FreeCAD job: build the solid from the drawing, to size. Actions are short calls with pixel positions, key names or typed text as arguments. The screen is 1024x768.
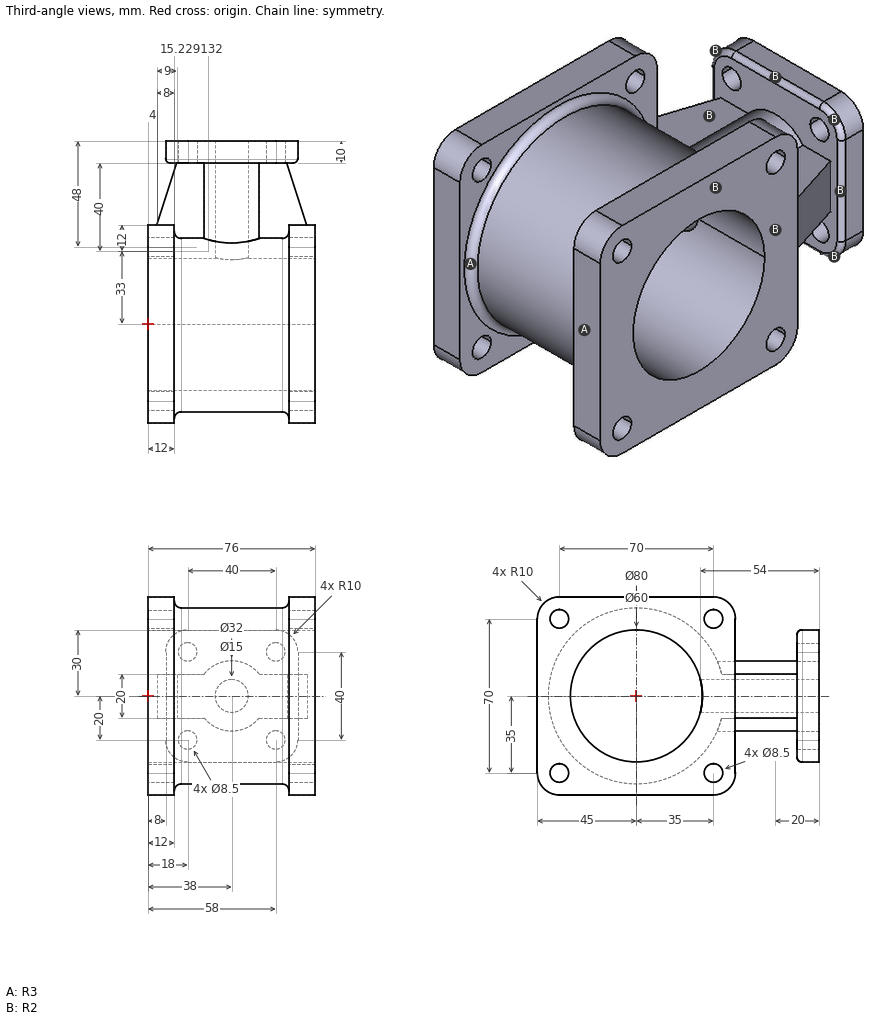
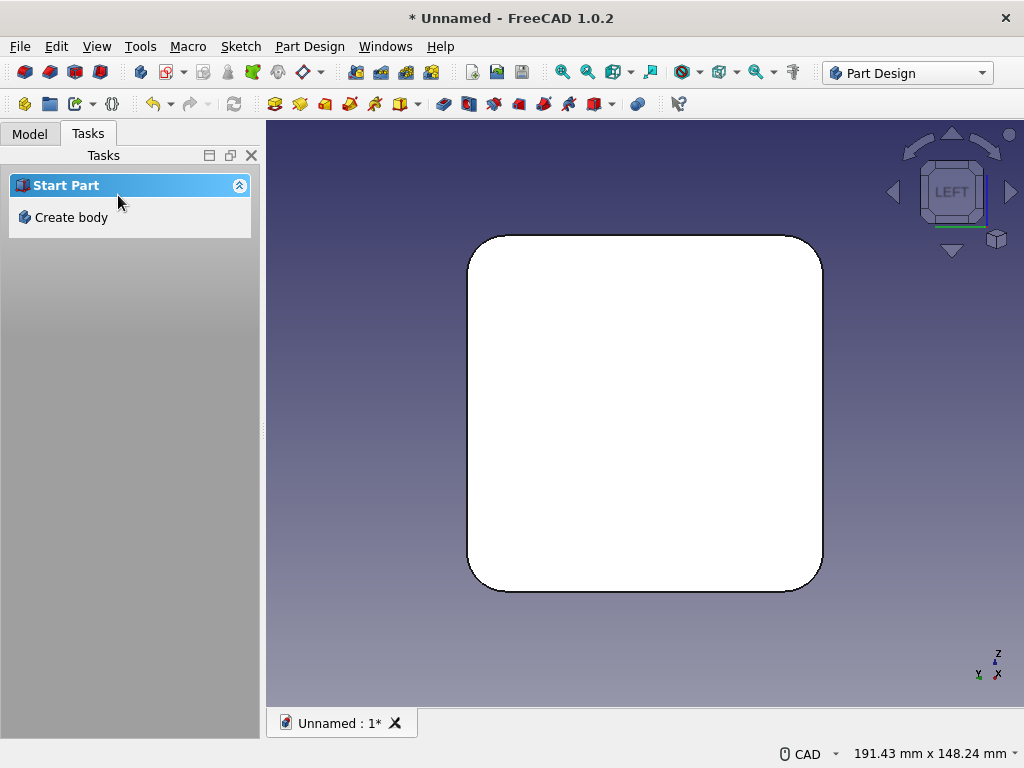
click(645, 412)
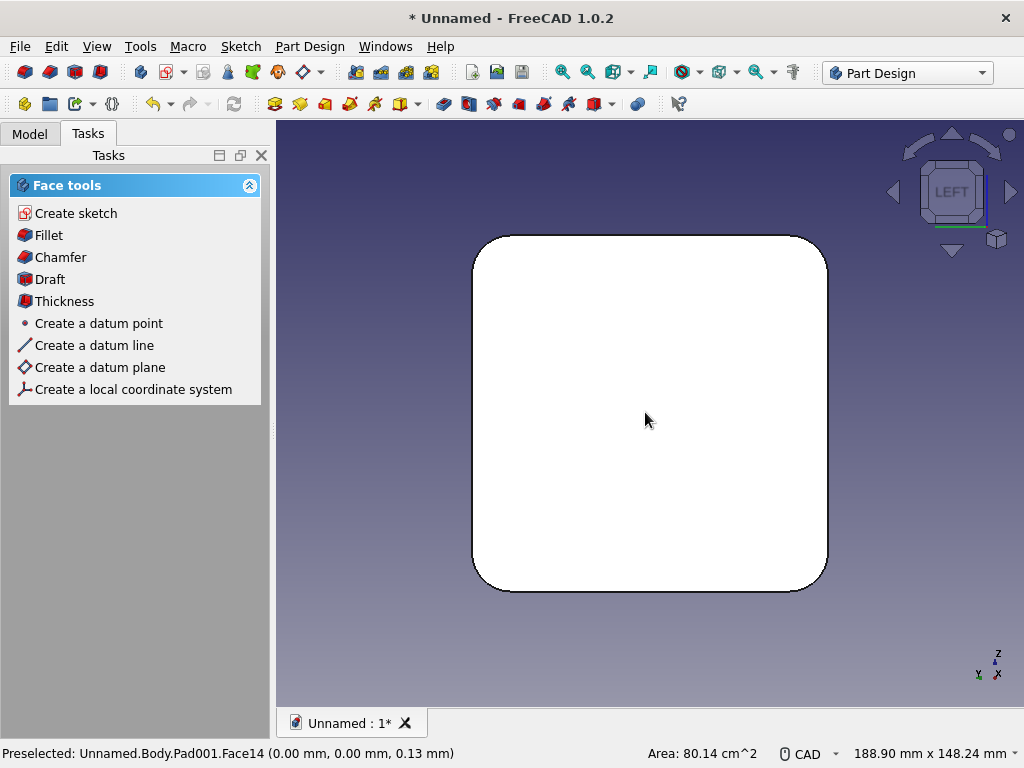
click(166, 72)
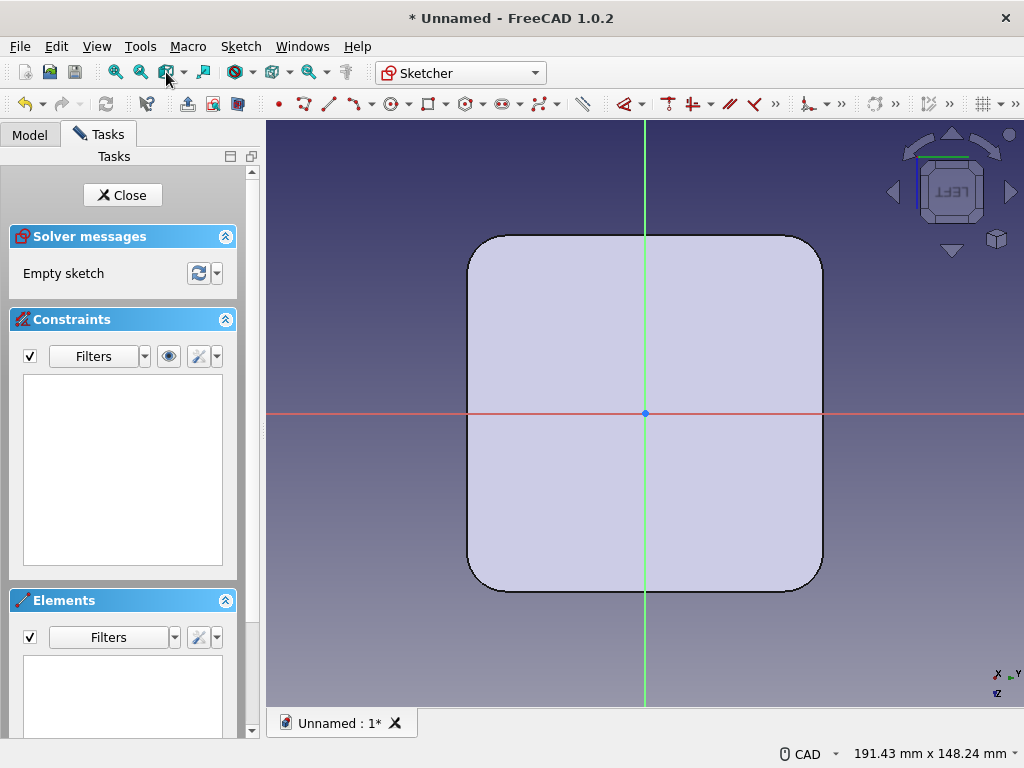
scroll(784, 413, up, 2)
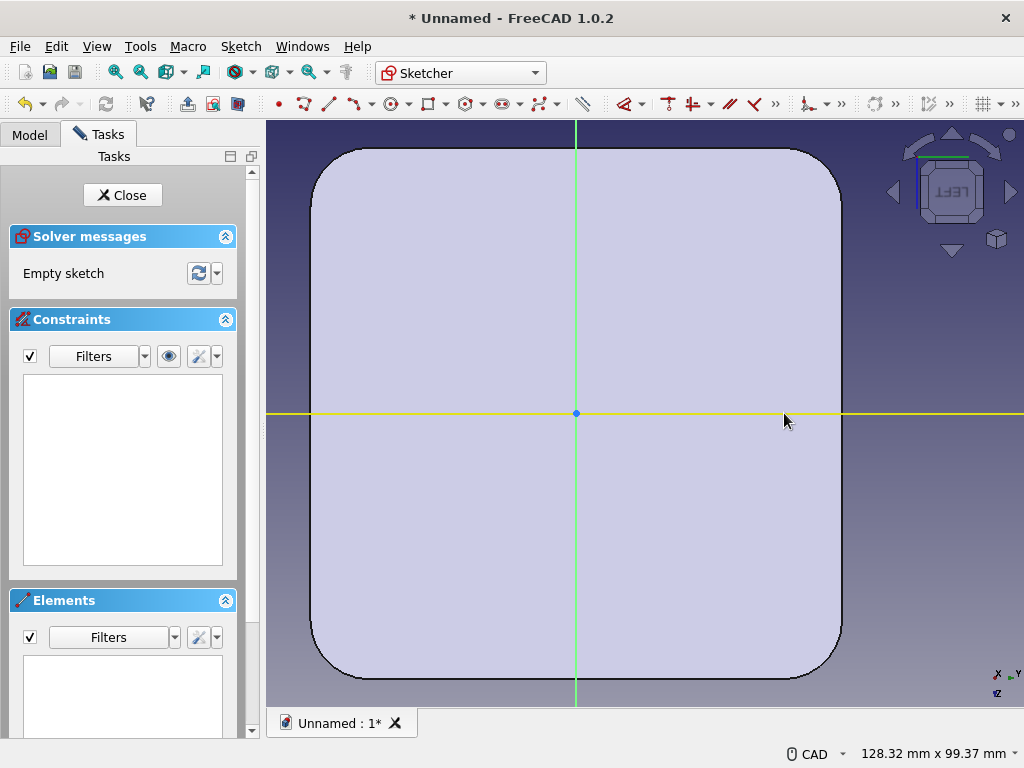
click(390, 104)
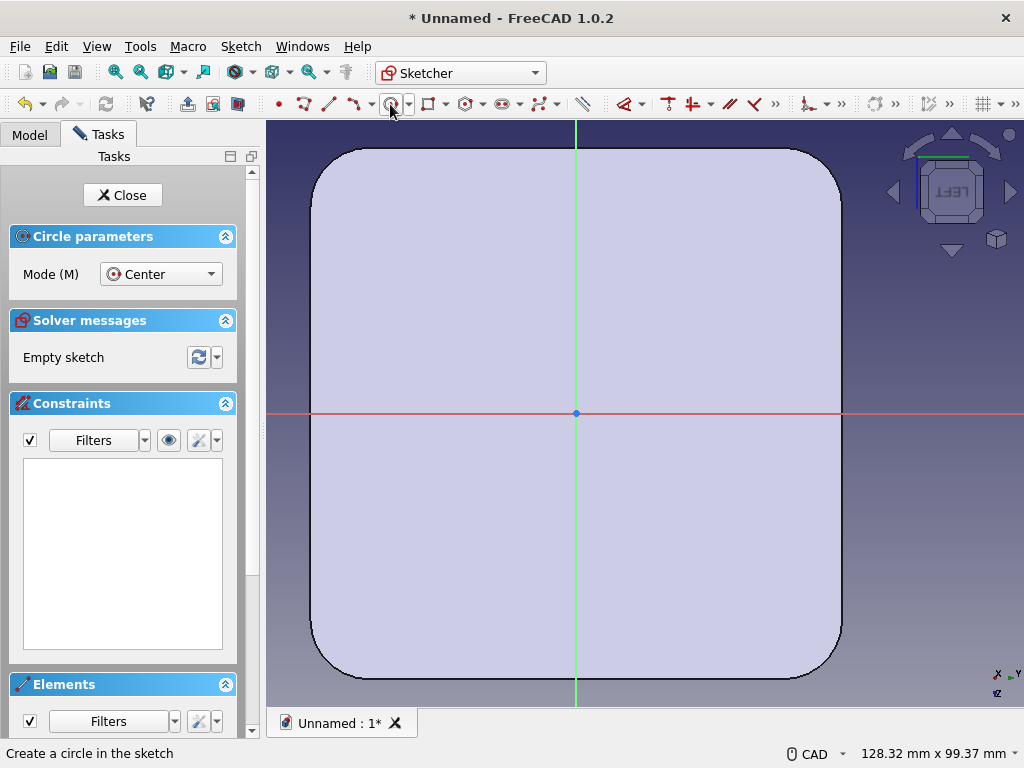
click(576, 414)
click(702, 288)
key(Escape)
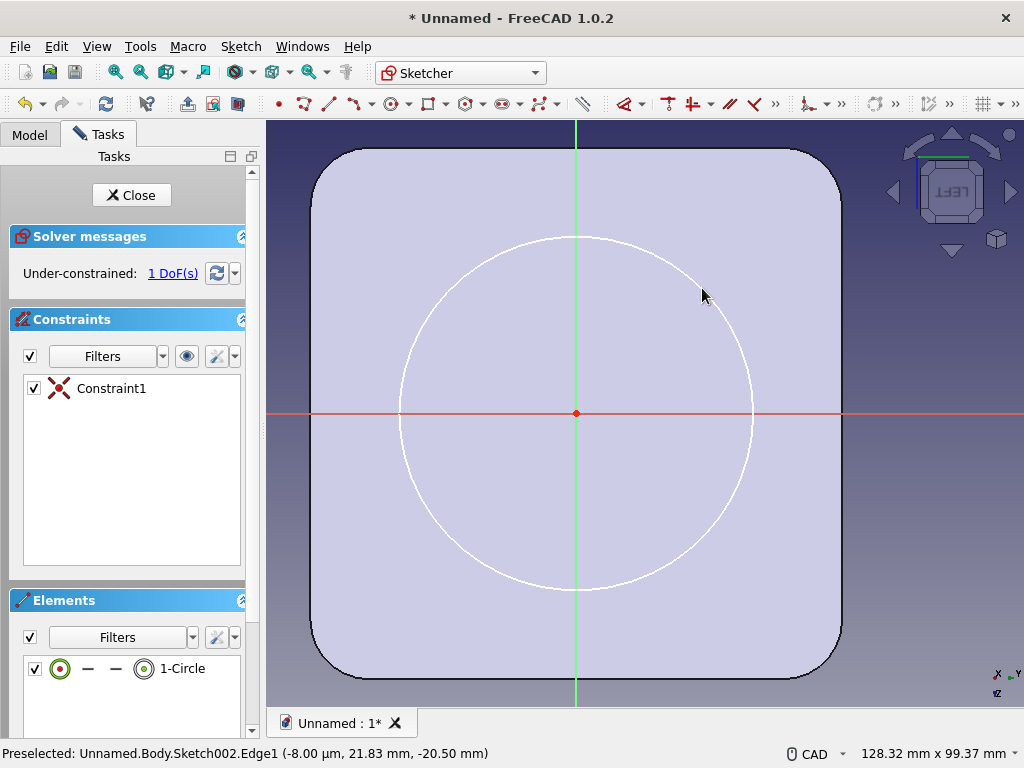
key(d)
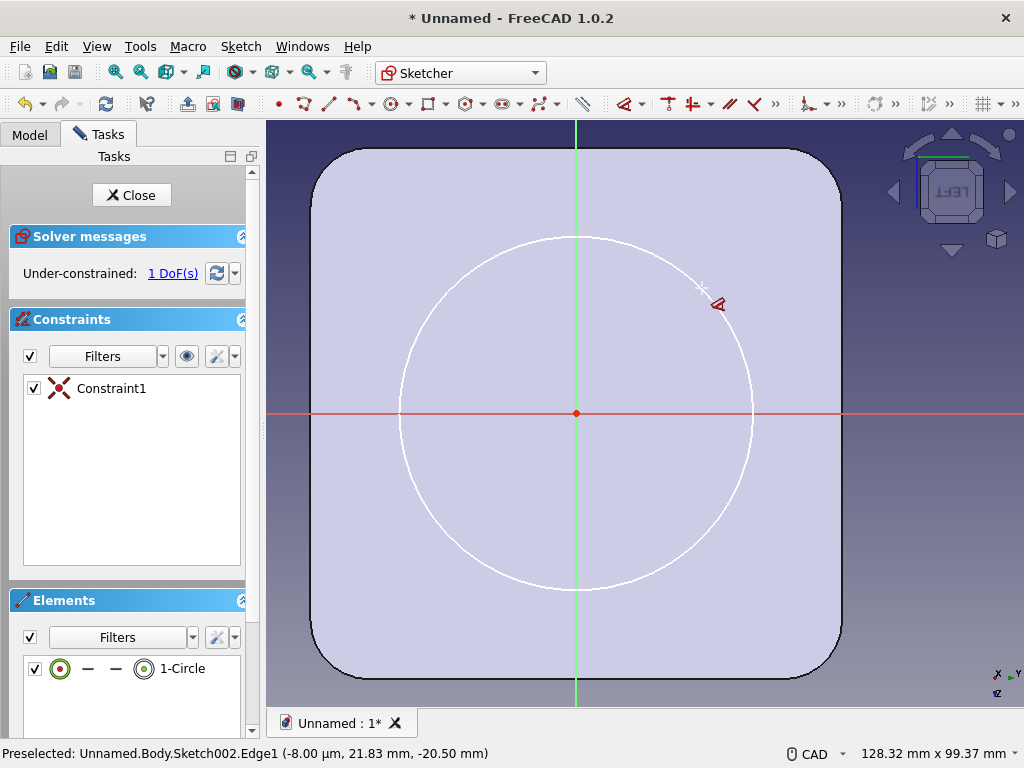
click(701, 288)
click(724, 265)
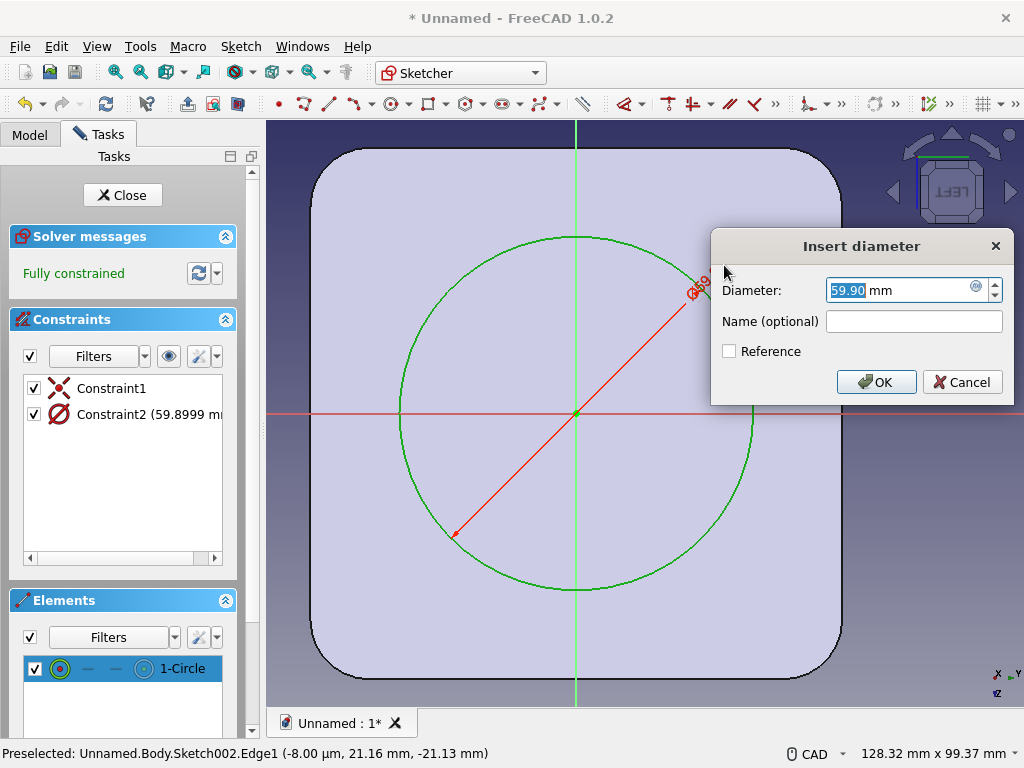
text(60)
key(Return)
key(Escape)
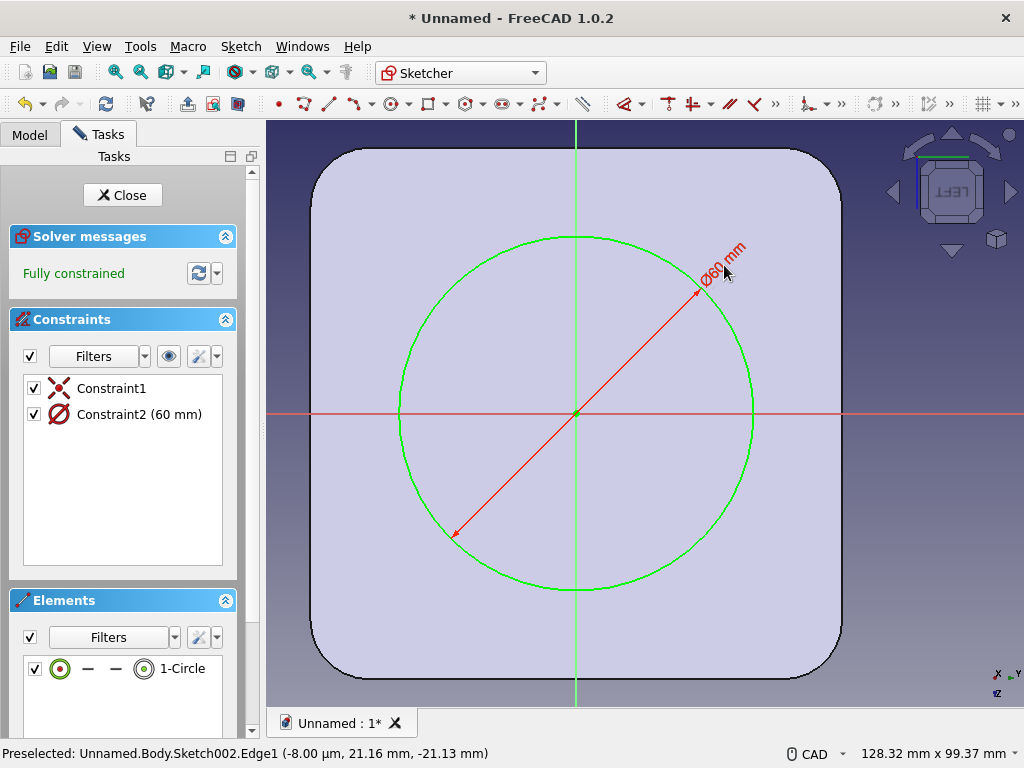
click(123, 195)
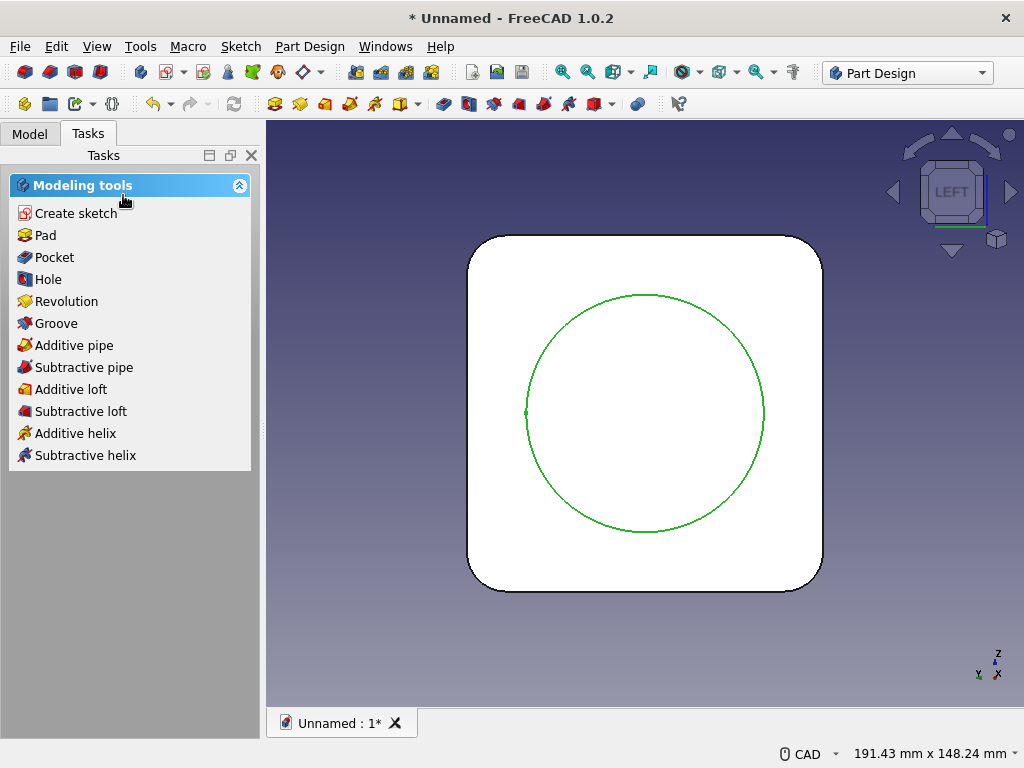
click(444, 104)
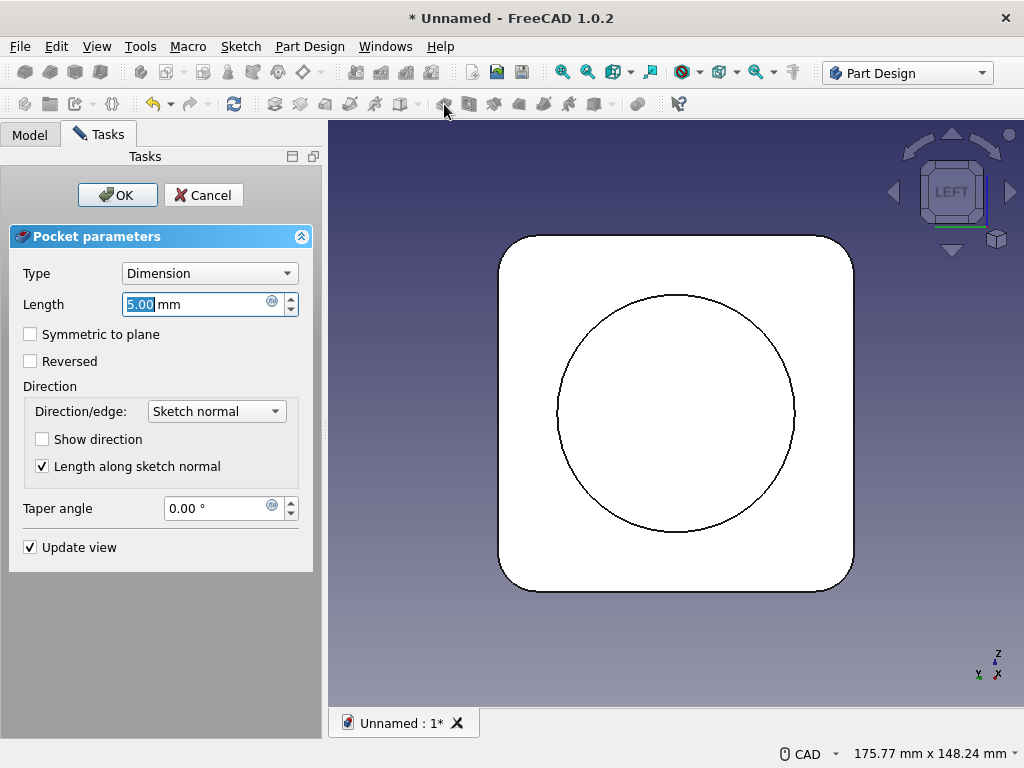
click(210, 274)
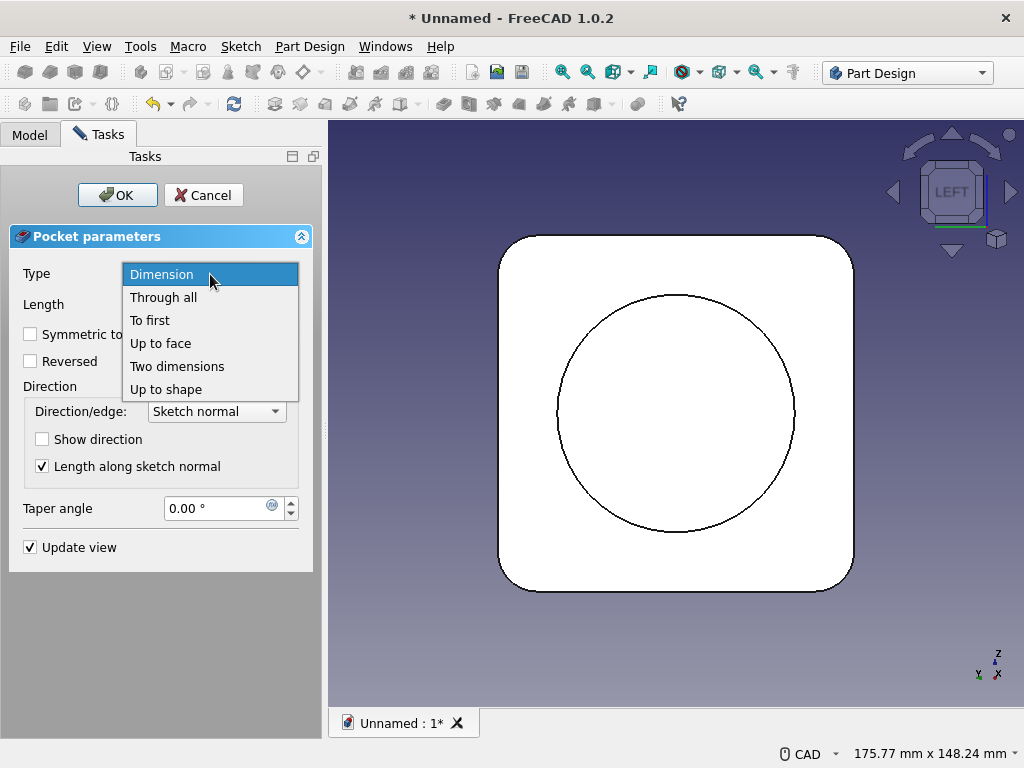
click(208, 298)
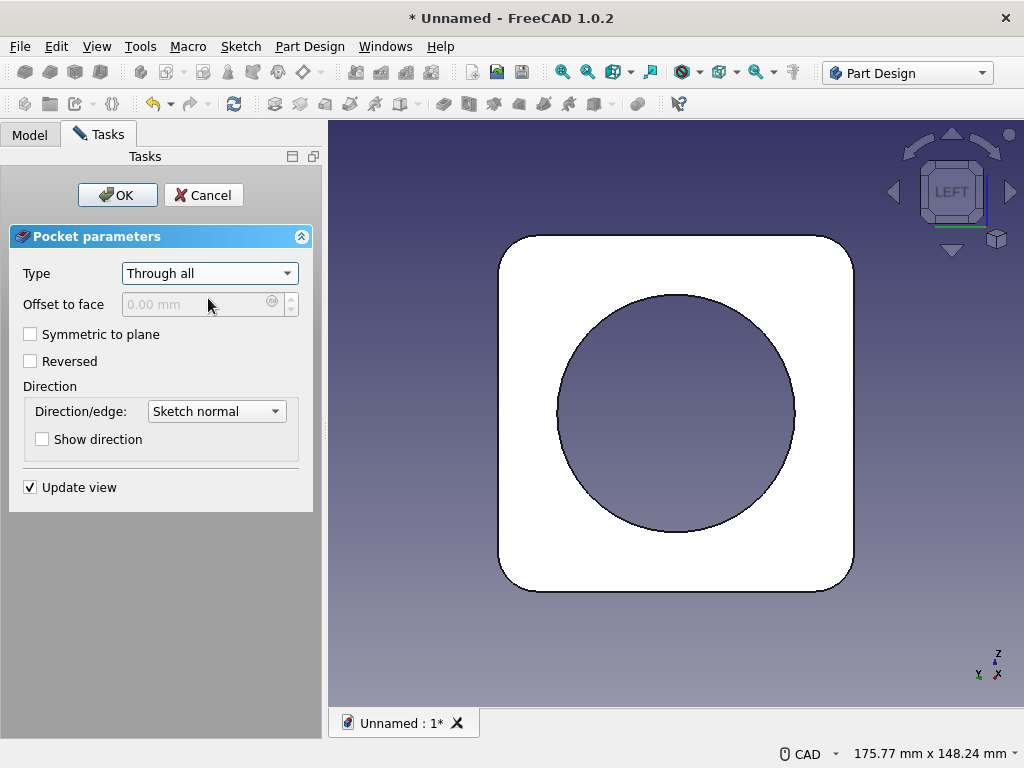
click(118, 195)